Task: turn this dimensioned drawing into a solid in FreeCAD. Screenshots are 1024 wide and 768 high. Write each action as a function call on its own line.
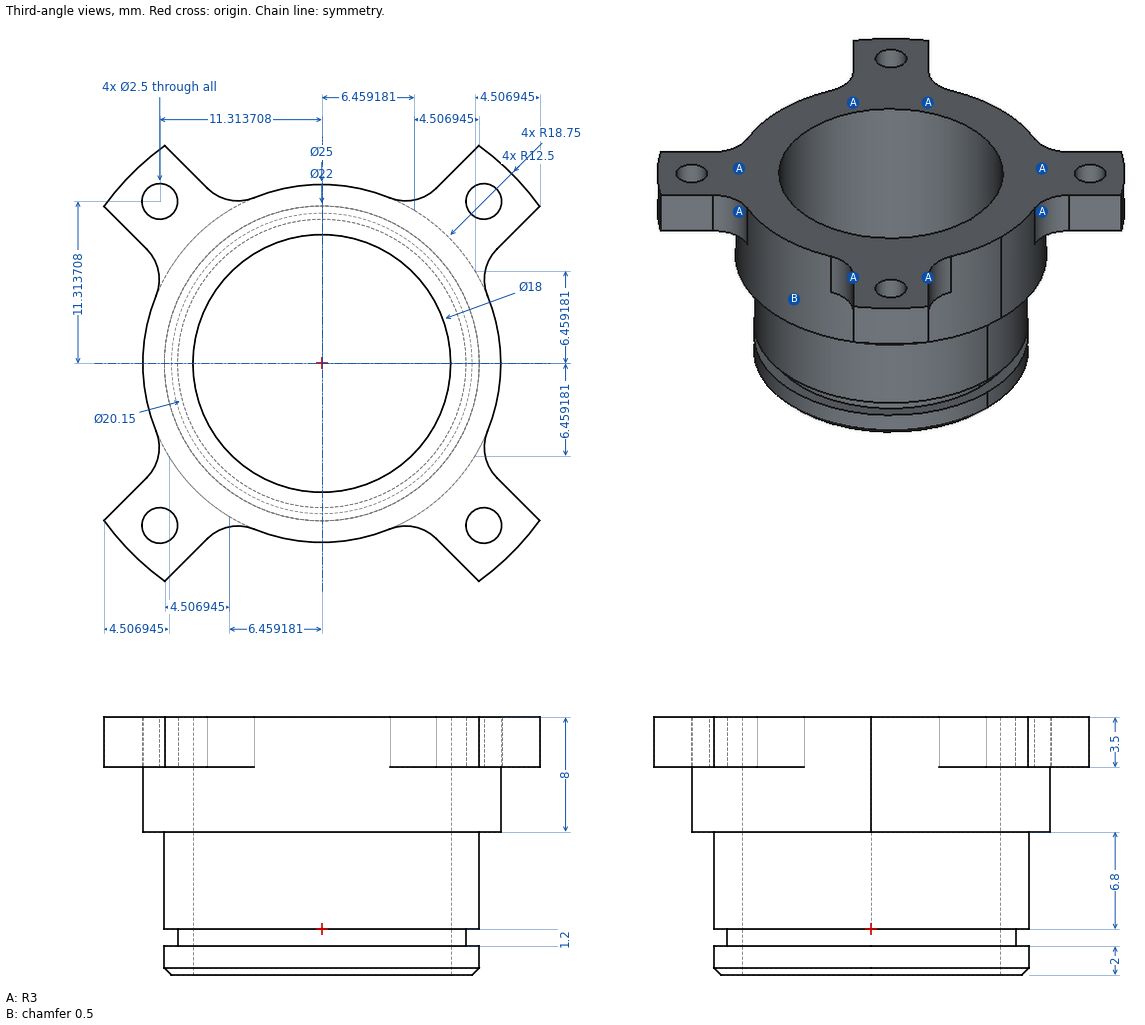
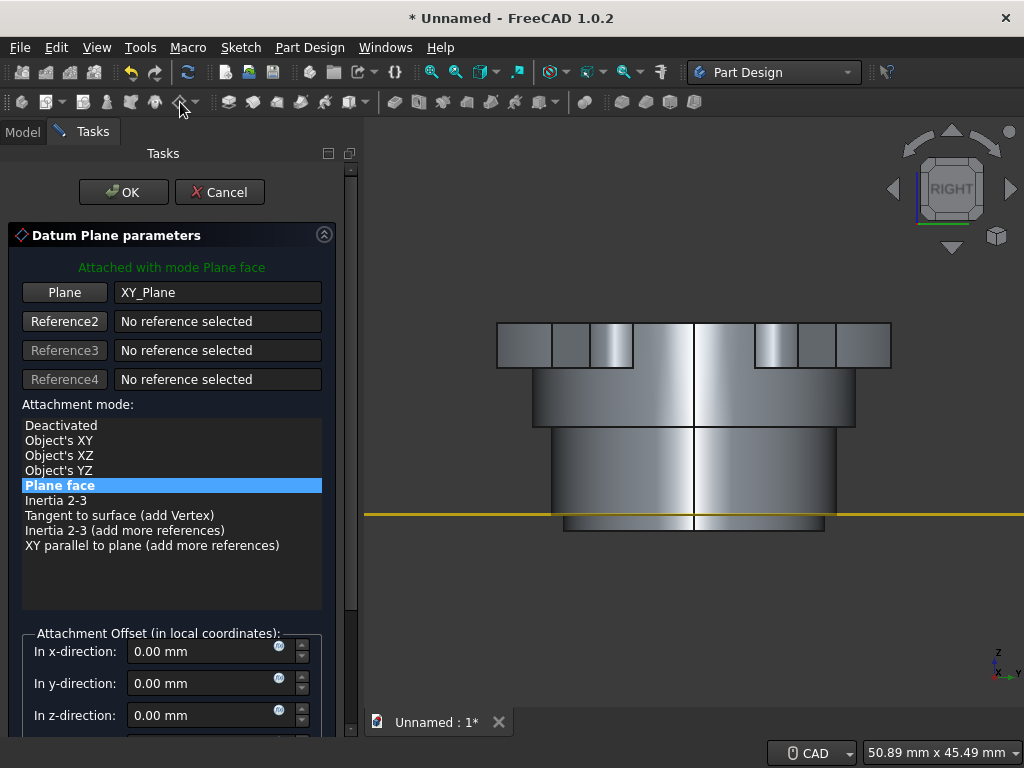
triple_click(210, 715)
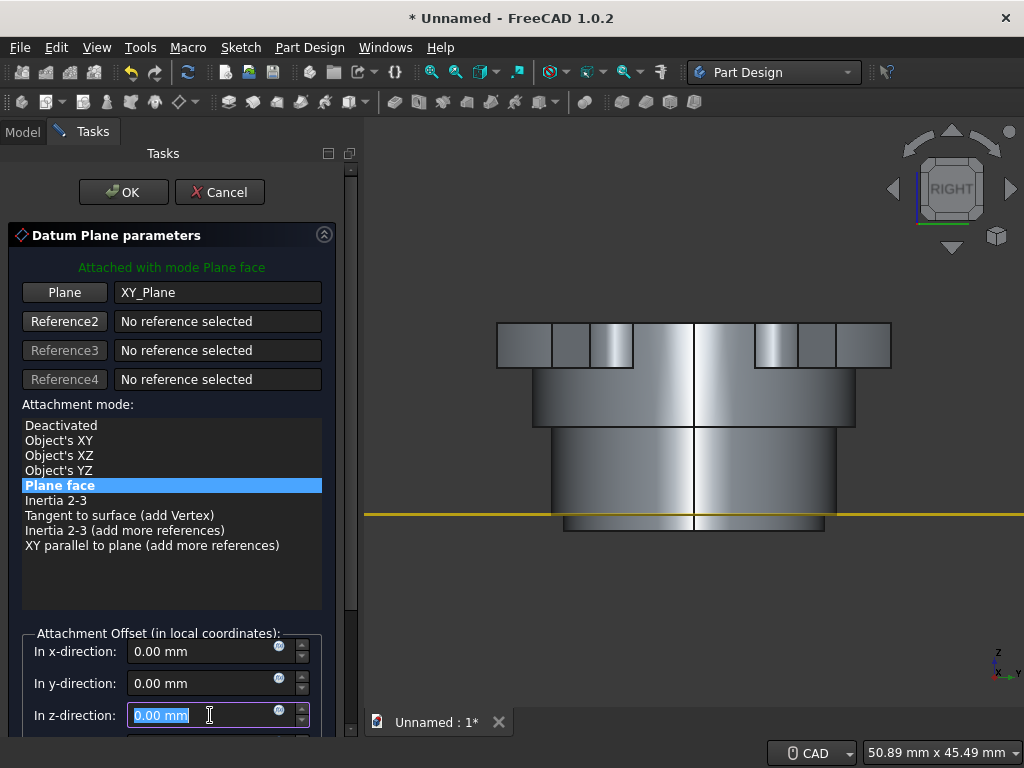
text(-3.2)
key(Tab)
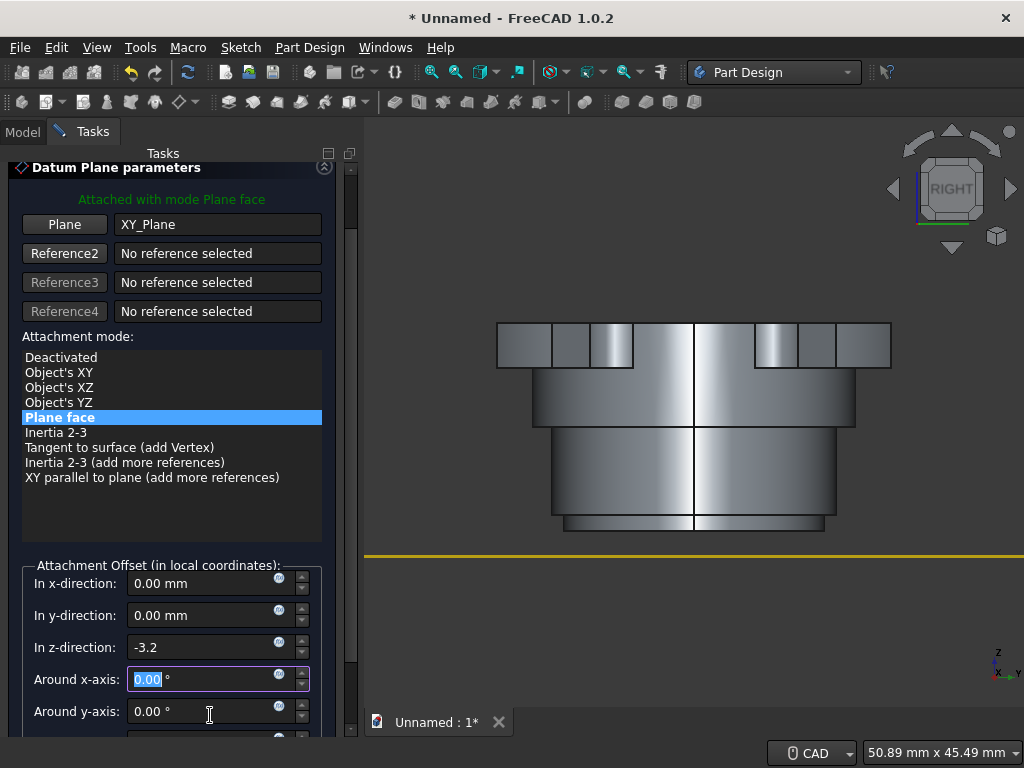
scroll(351, 450, up, 2)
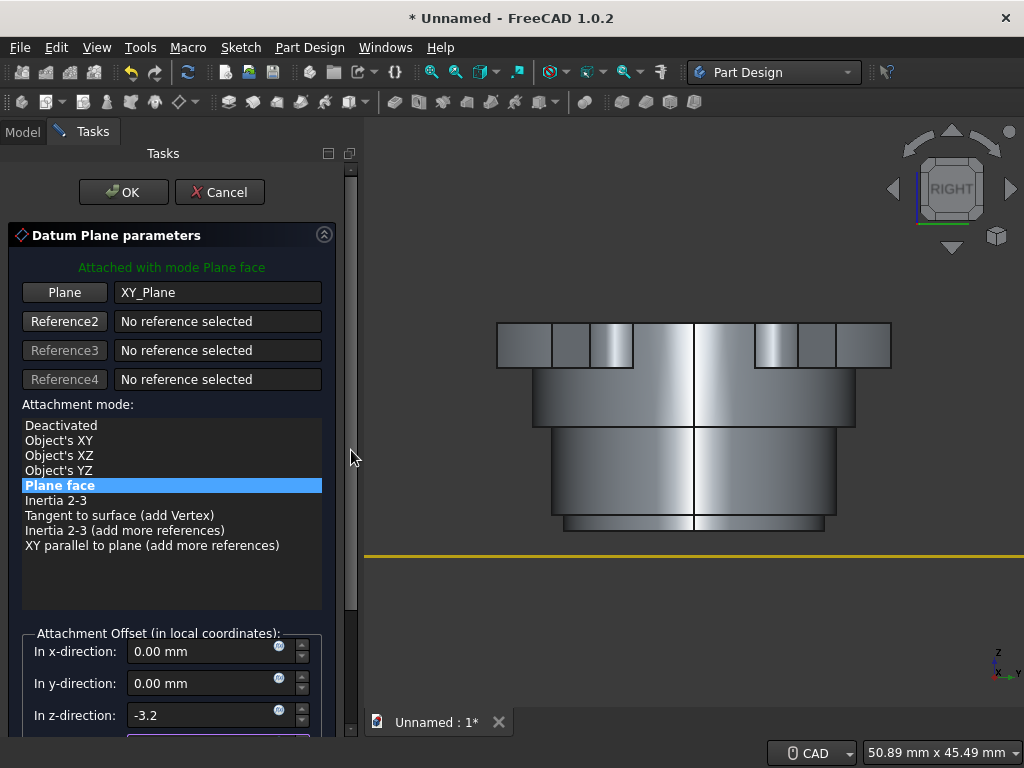
click(124, 192)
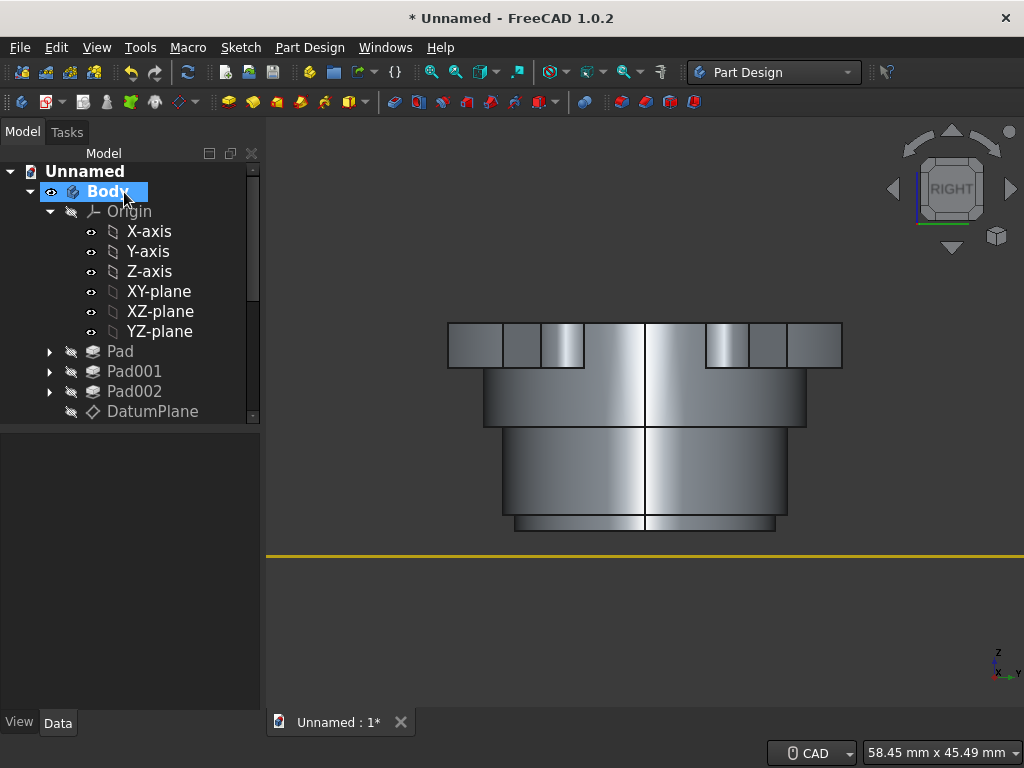
scroll(100, 287, down, 3)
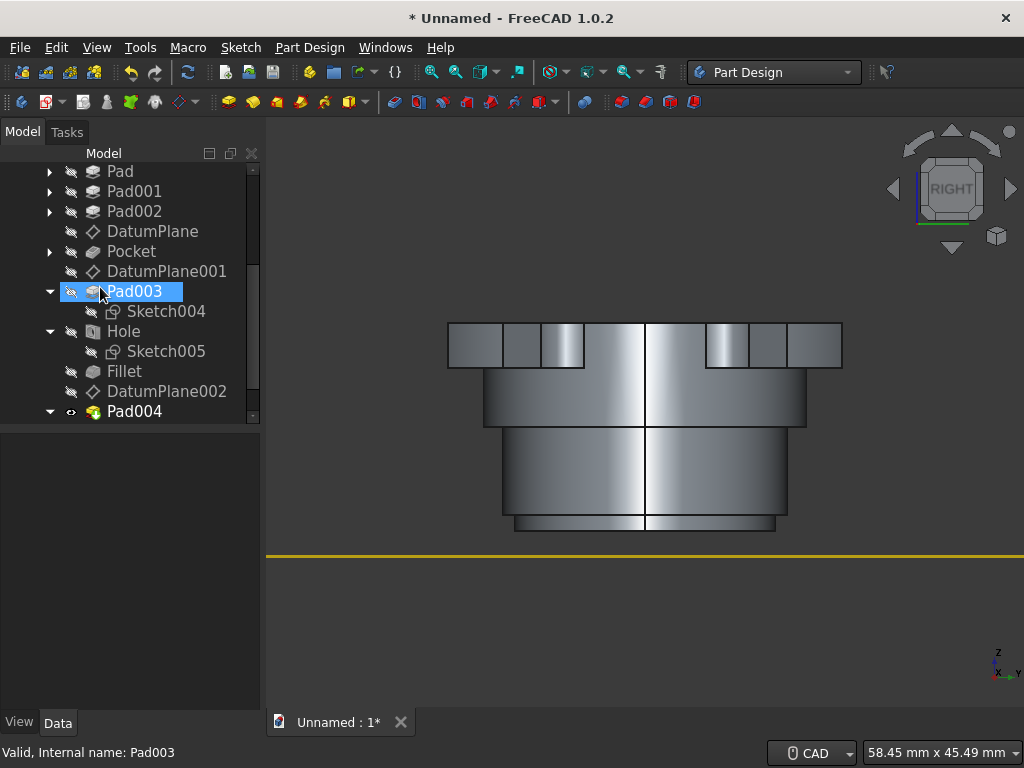
scroll(140, 287, up, 15)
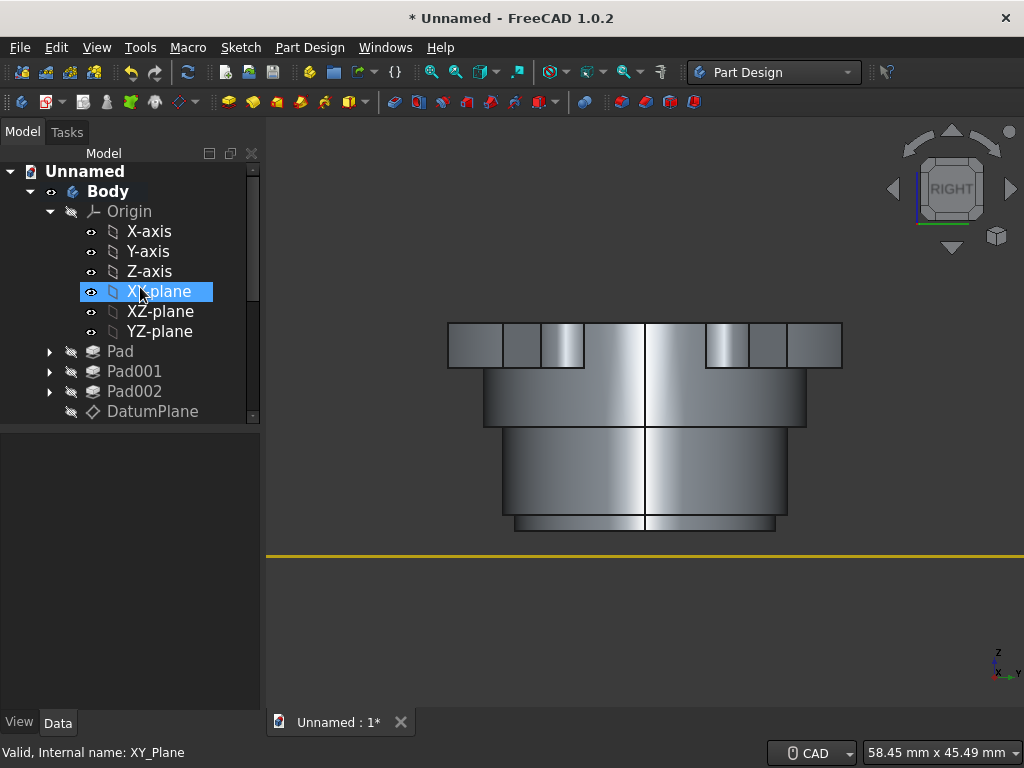
scroll(100, 287, down, 6)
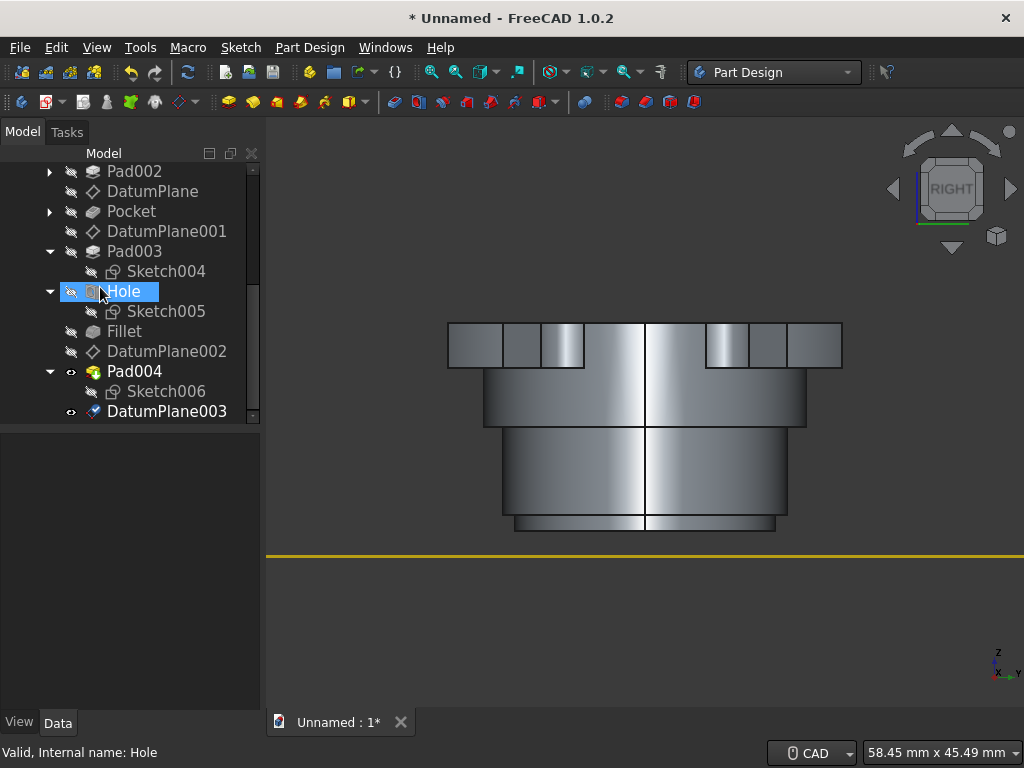
click(116, 412)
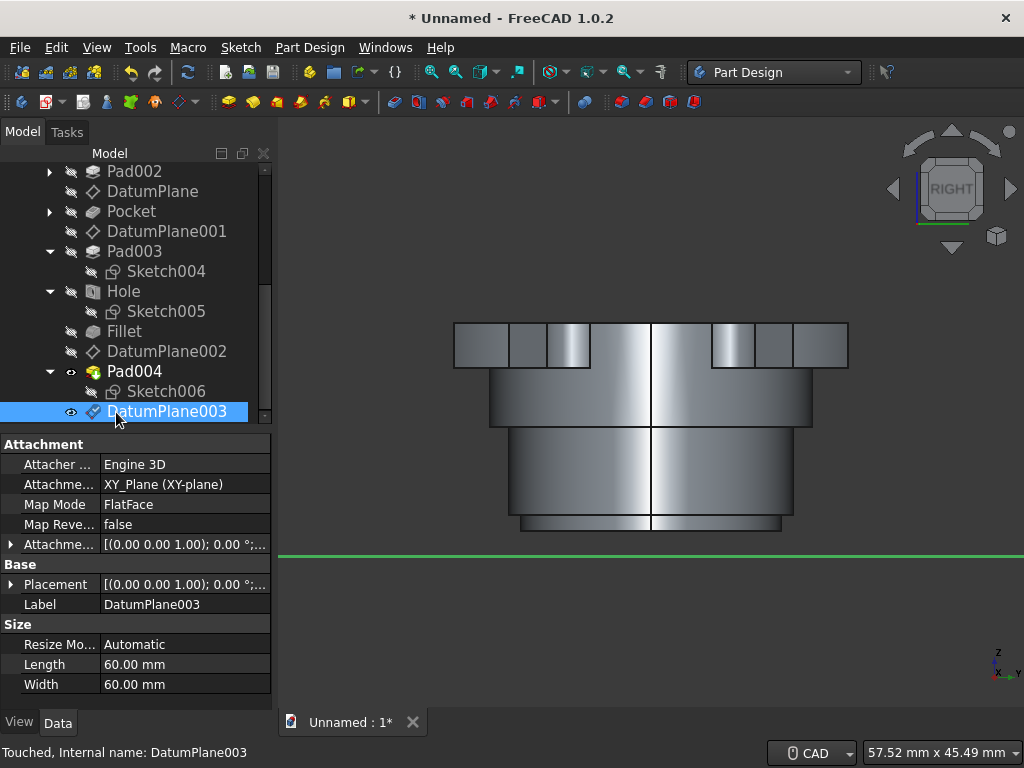
click(46, 102)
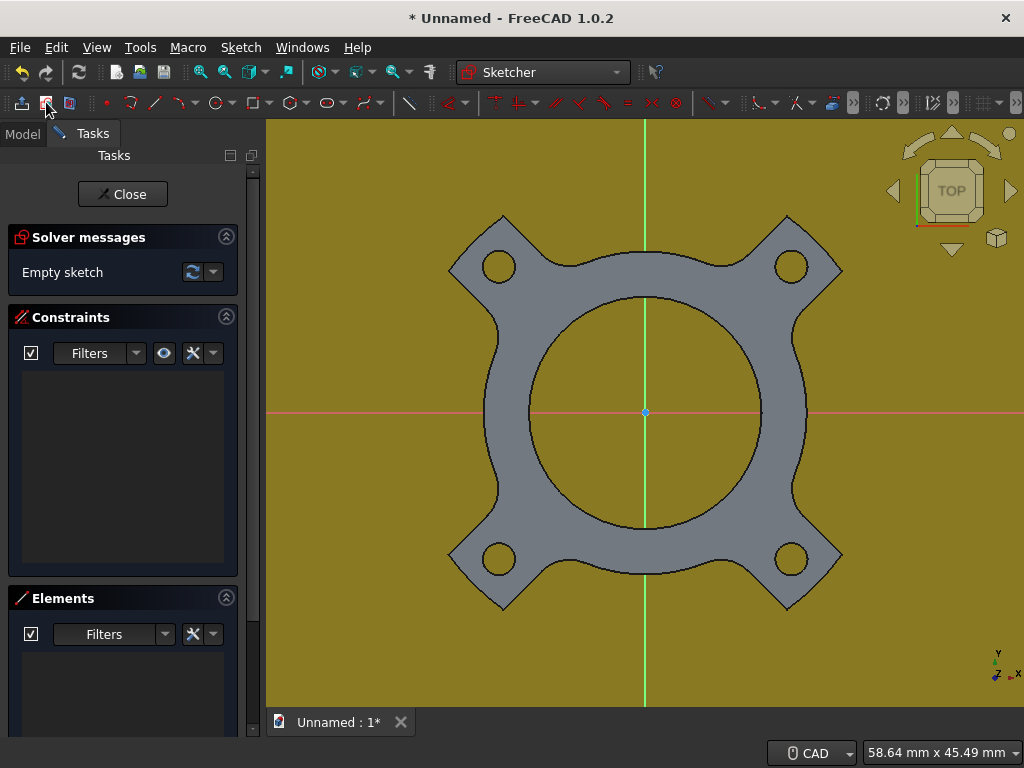
click(70, 104)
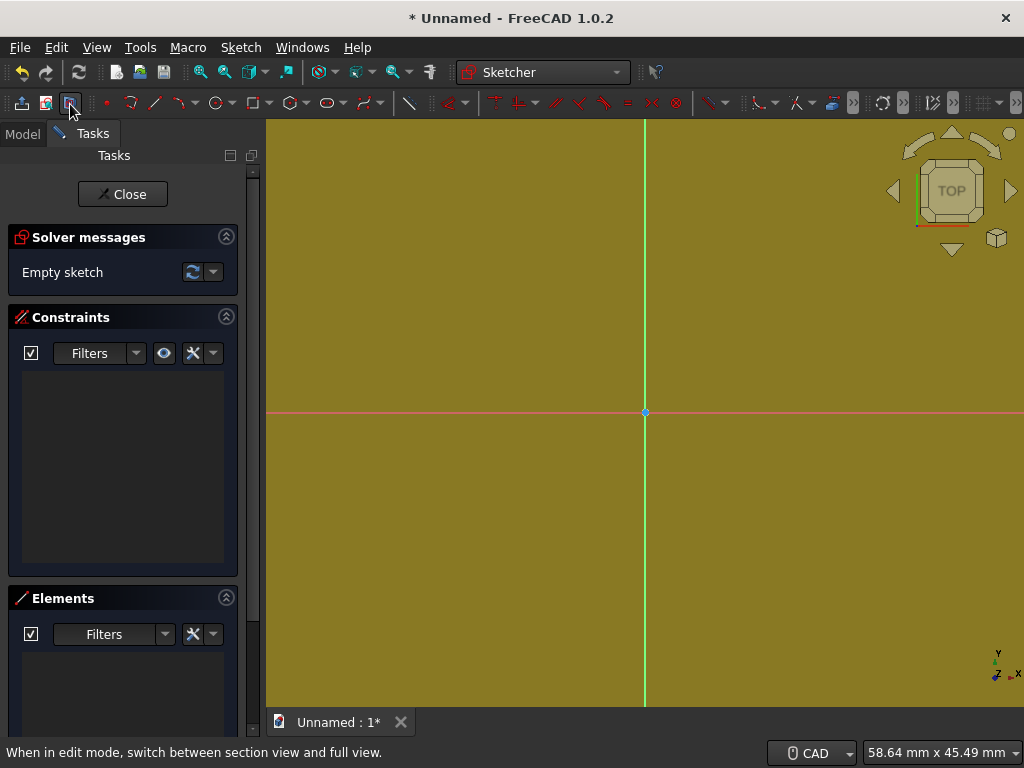
click(216, 104)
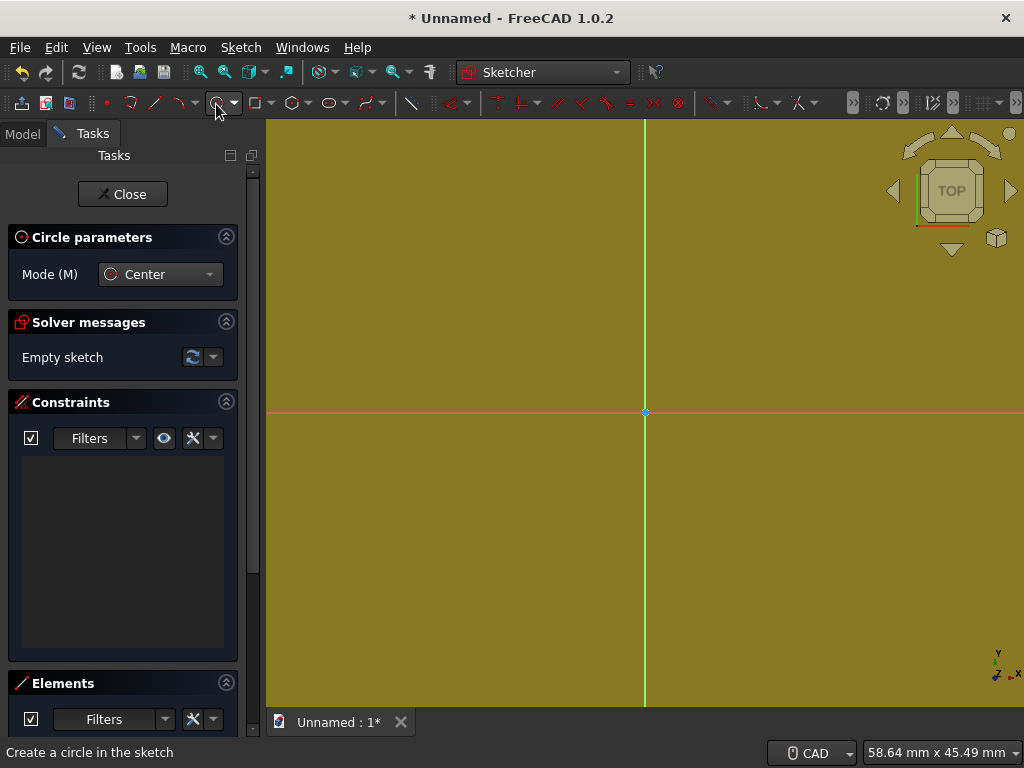
click(645, 413)
click(746, 312)